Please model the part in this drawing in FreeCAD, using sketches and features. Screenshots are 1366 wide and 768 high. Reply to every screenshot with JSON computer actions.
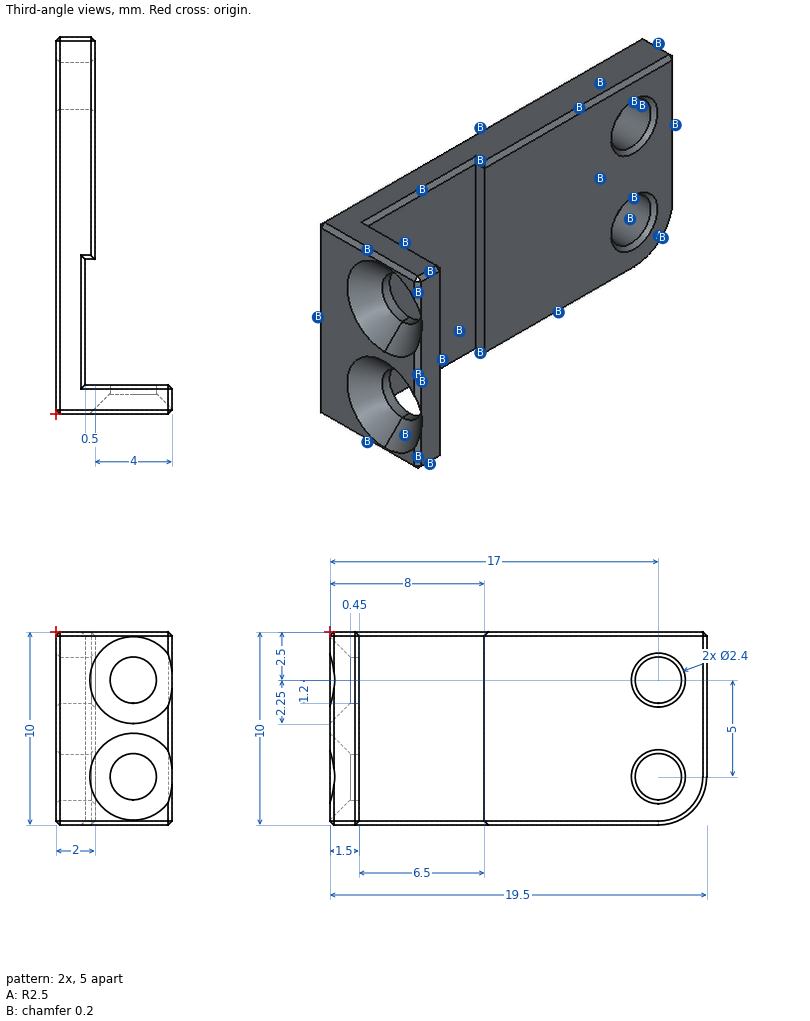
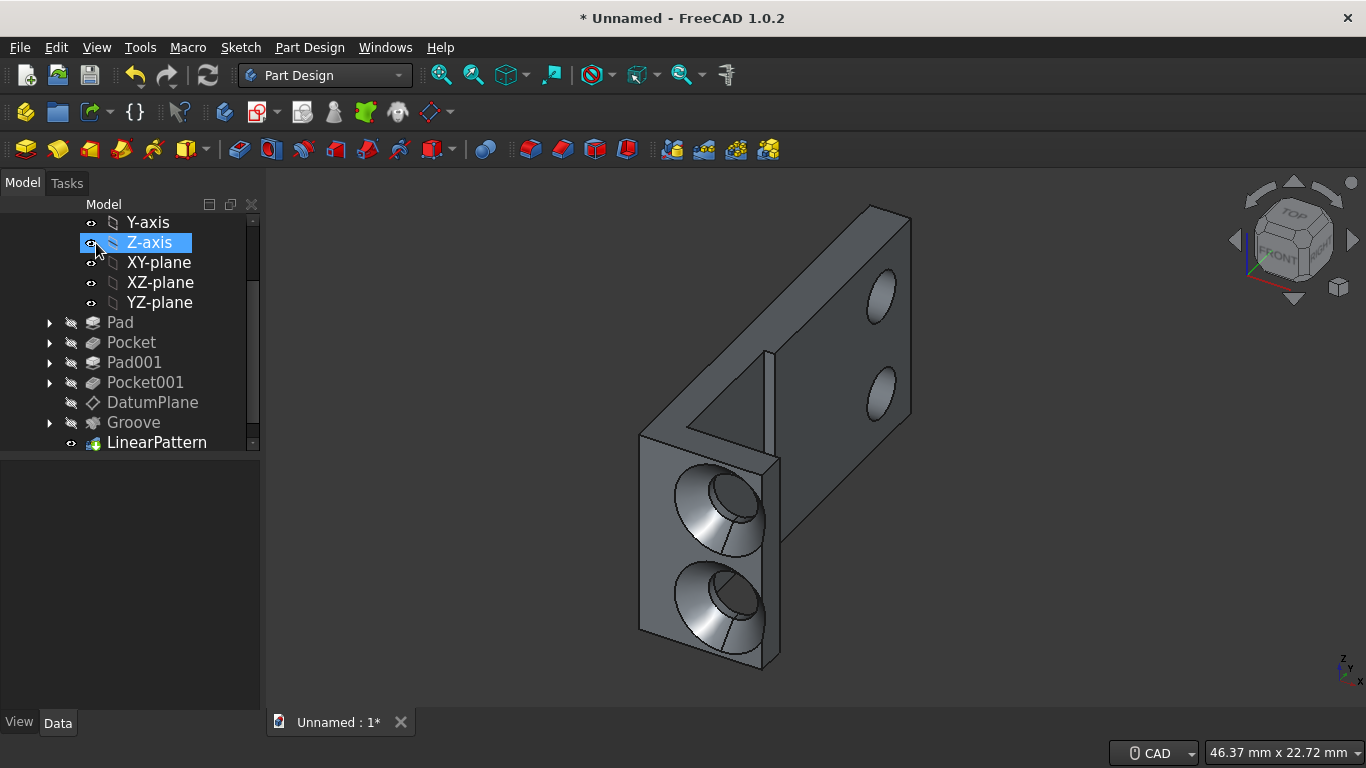
{"action": "key", "text": "0"}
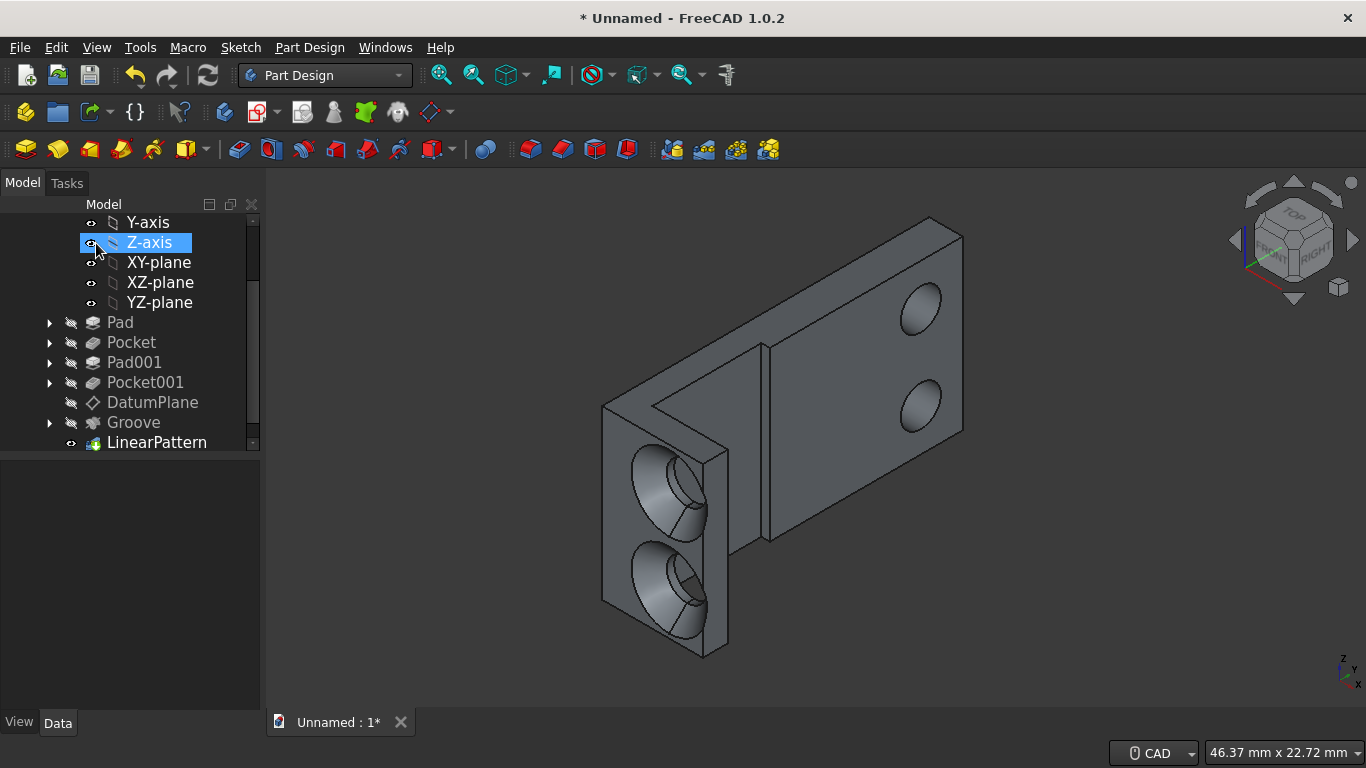
{"action": "key", "text": "2"}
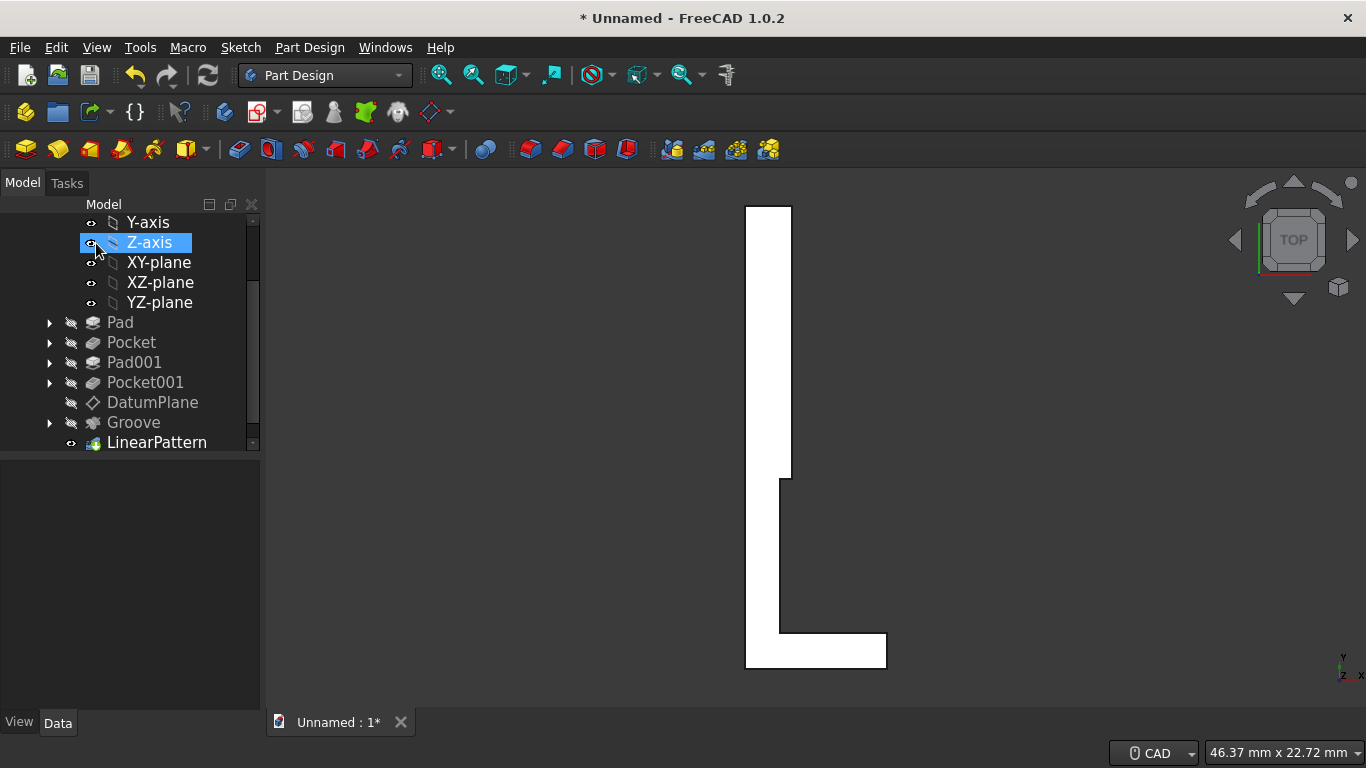
{"action": "key", "text": "1"}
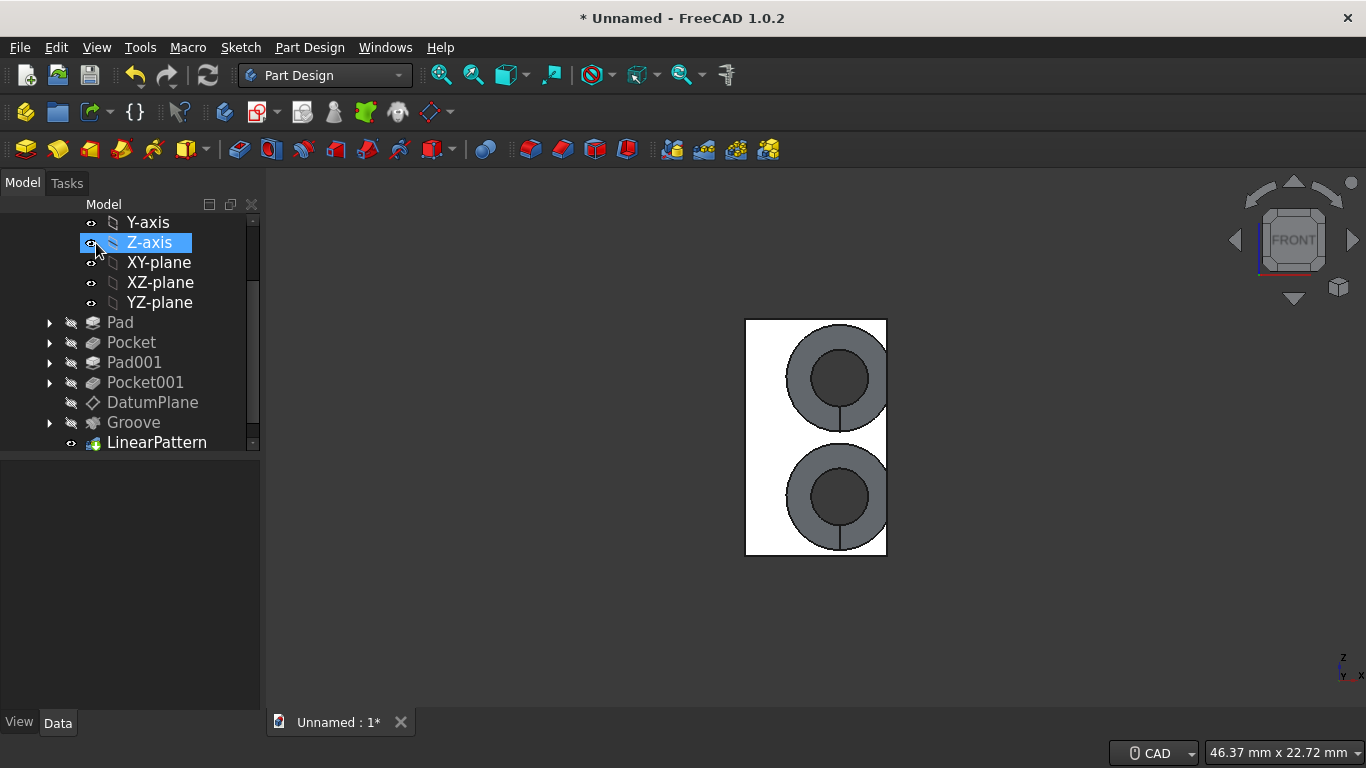
{"action": "left_click", "coordinate": [442, 76]}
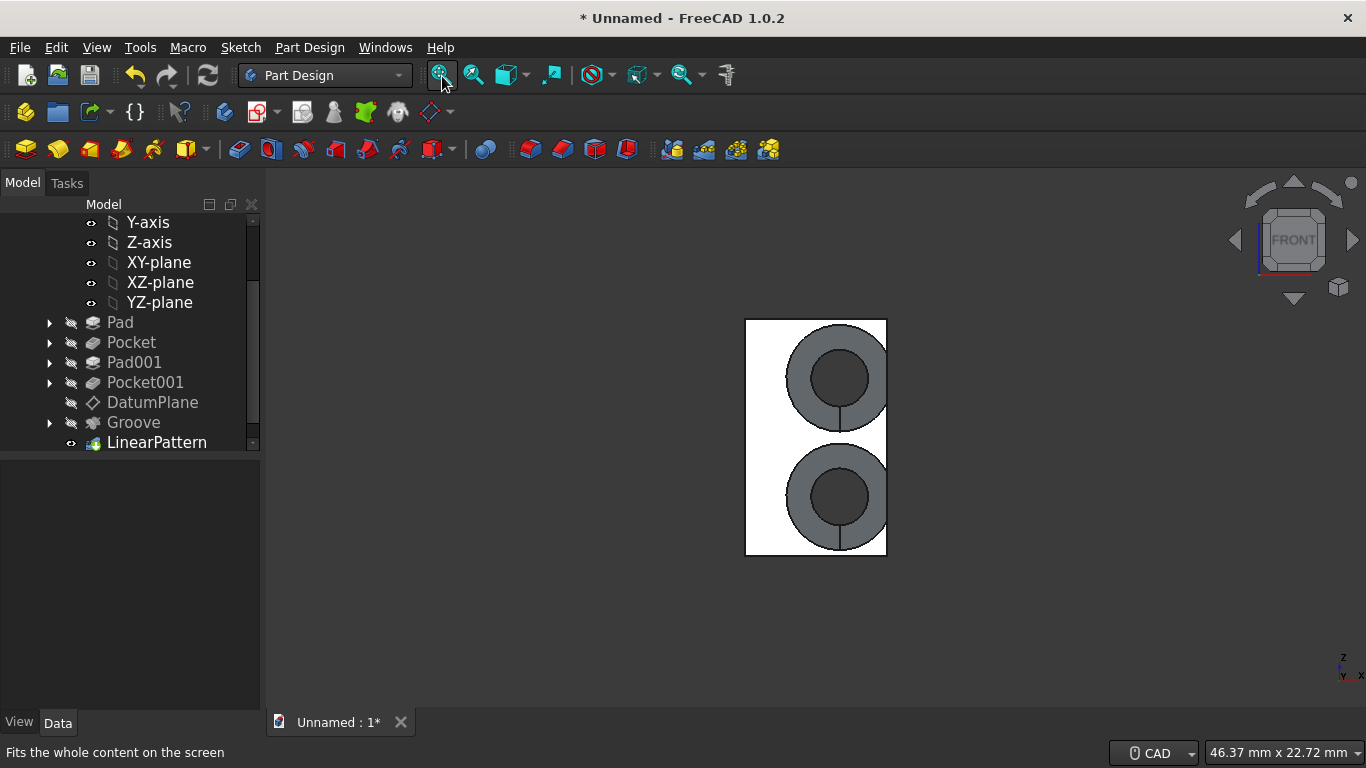
{"action": "key", "text": "3"}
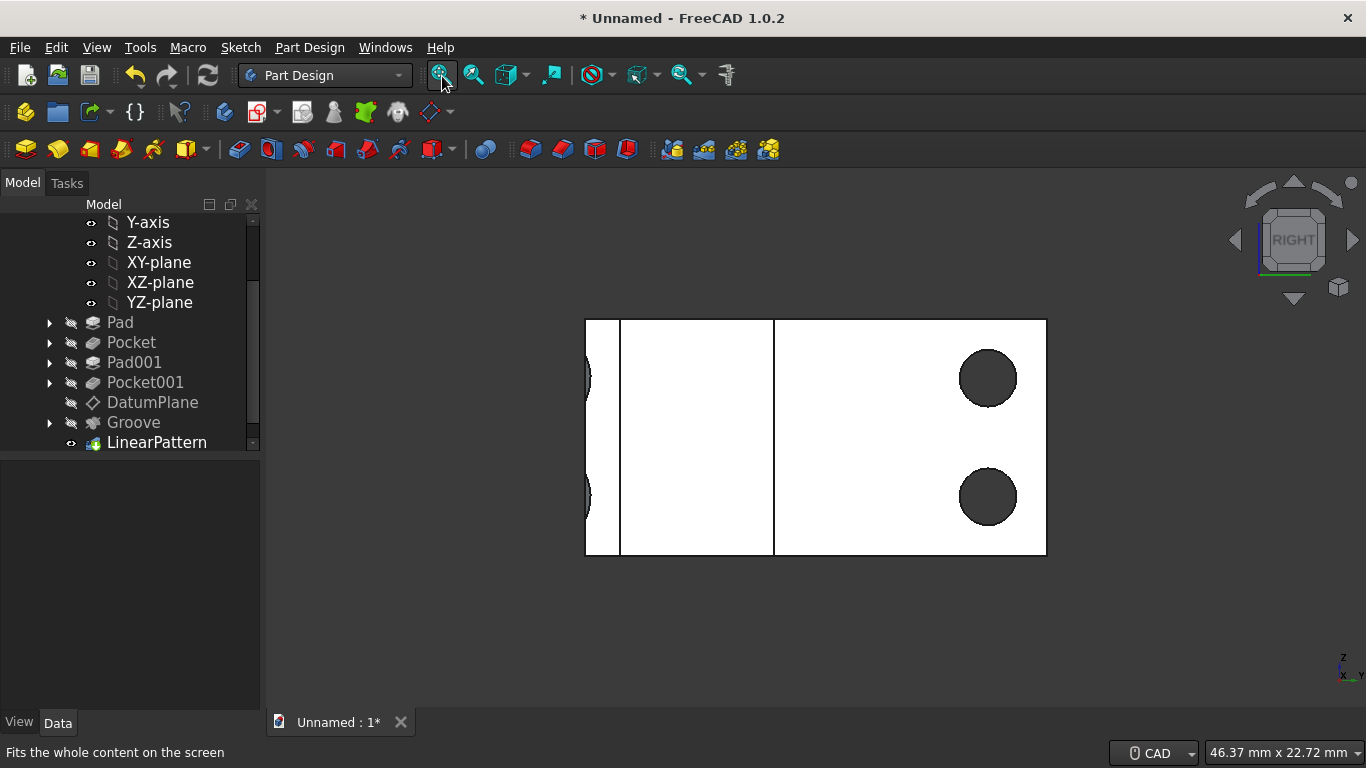
{"action": "left_click", "coordinate": [442, 76]}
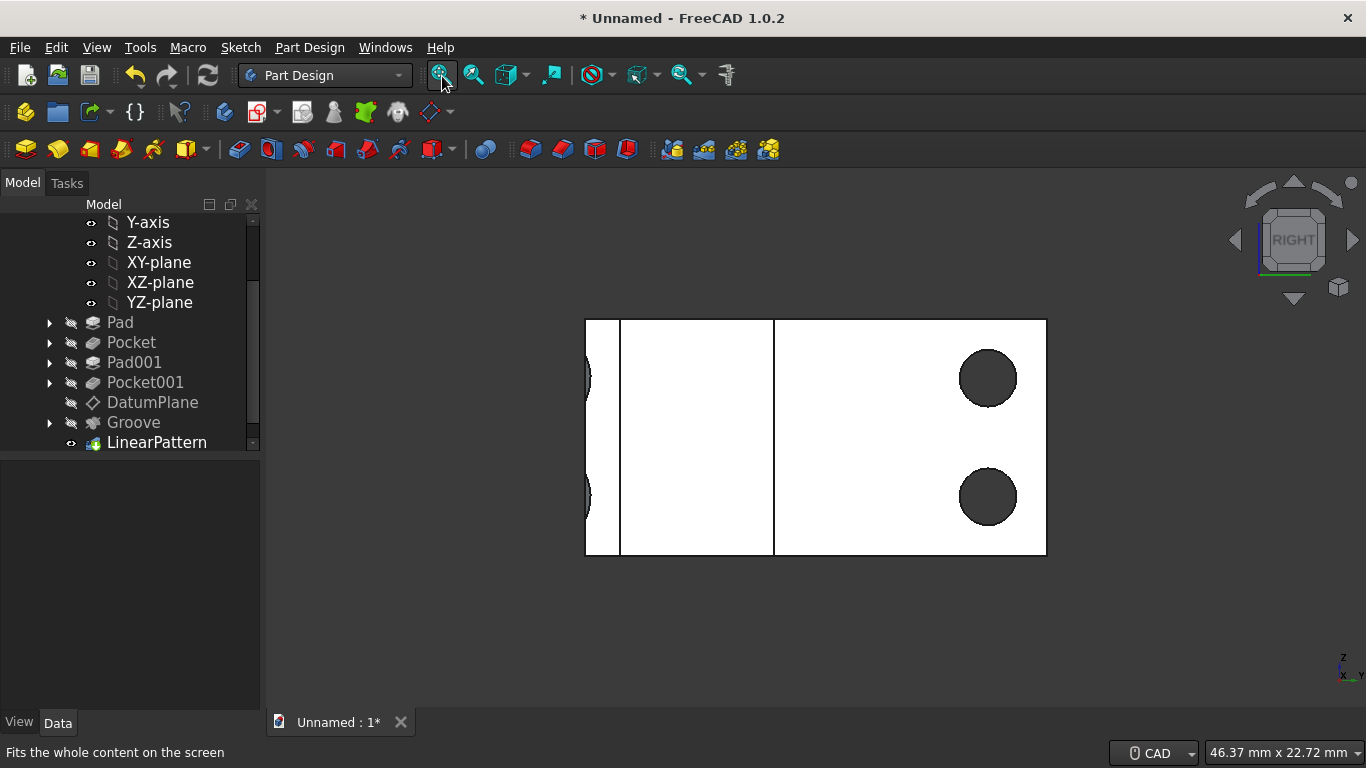
{"action": "key", "text": "5"}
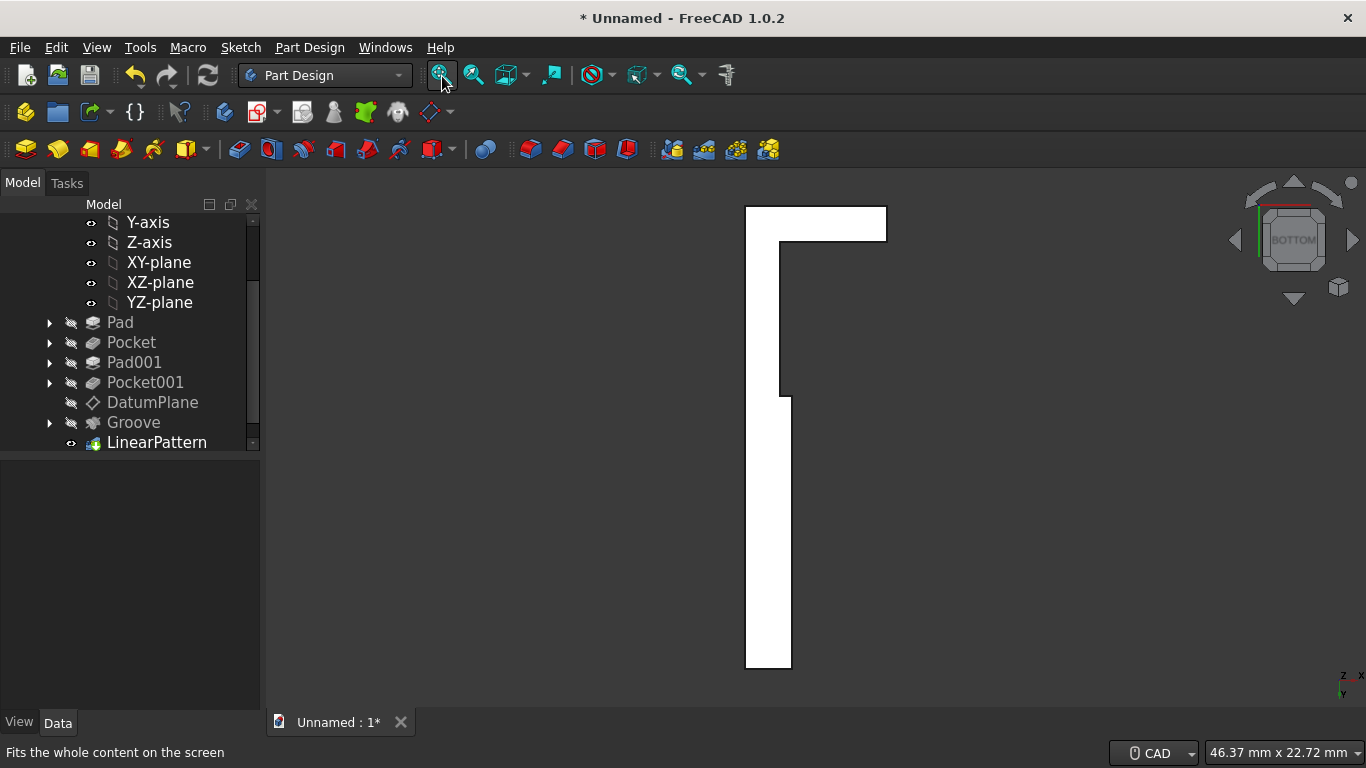
{"action": "key", "text": "4"}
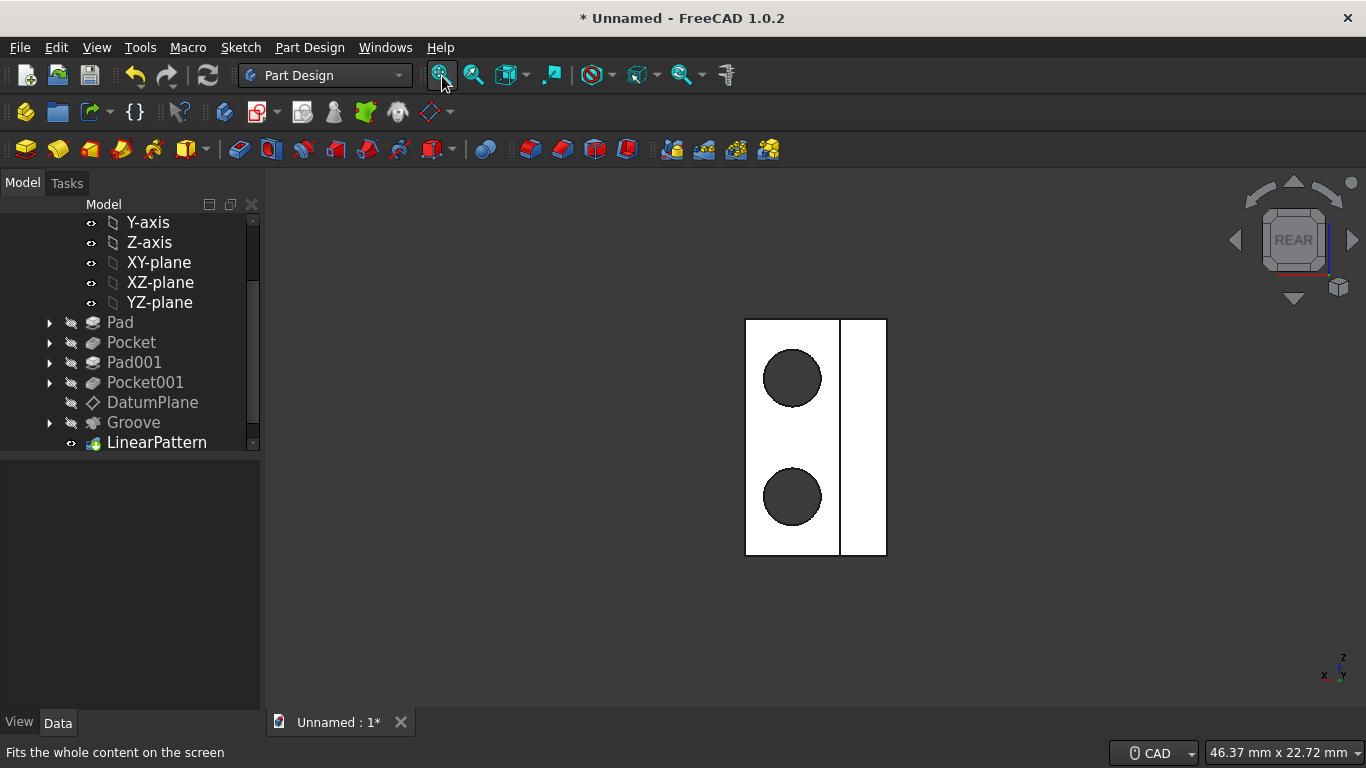
{"action": "left_click", "coordinate": [442, 76]}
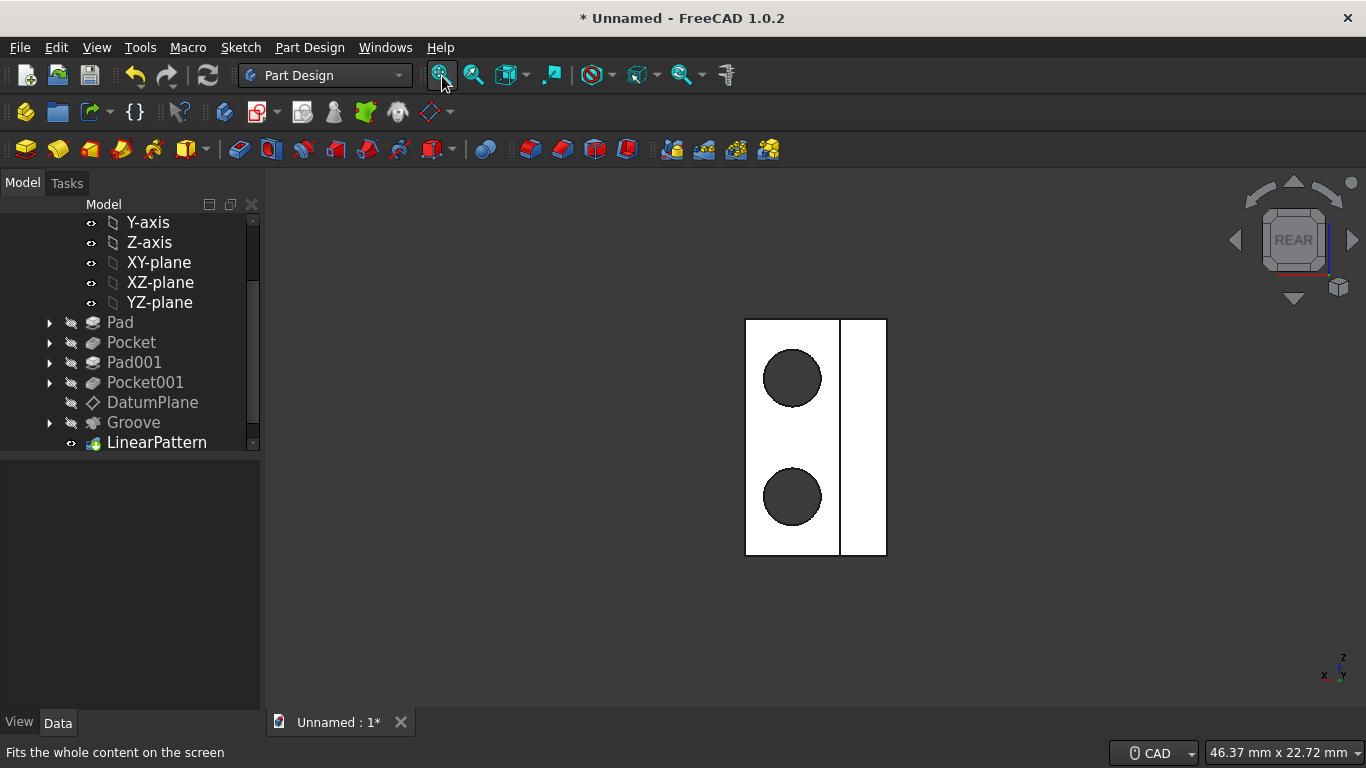
{"action": "left_click", "coordinate": [863, 555]}